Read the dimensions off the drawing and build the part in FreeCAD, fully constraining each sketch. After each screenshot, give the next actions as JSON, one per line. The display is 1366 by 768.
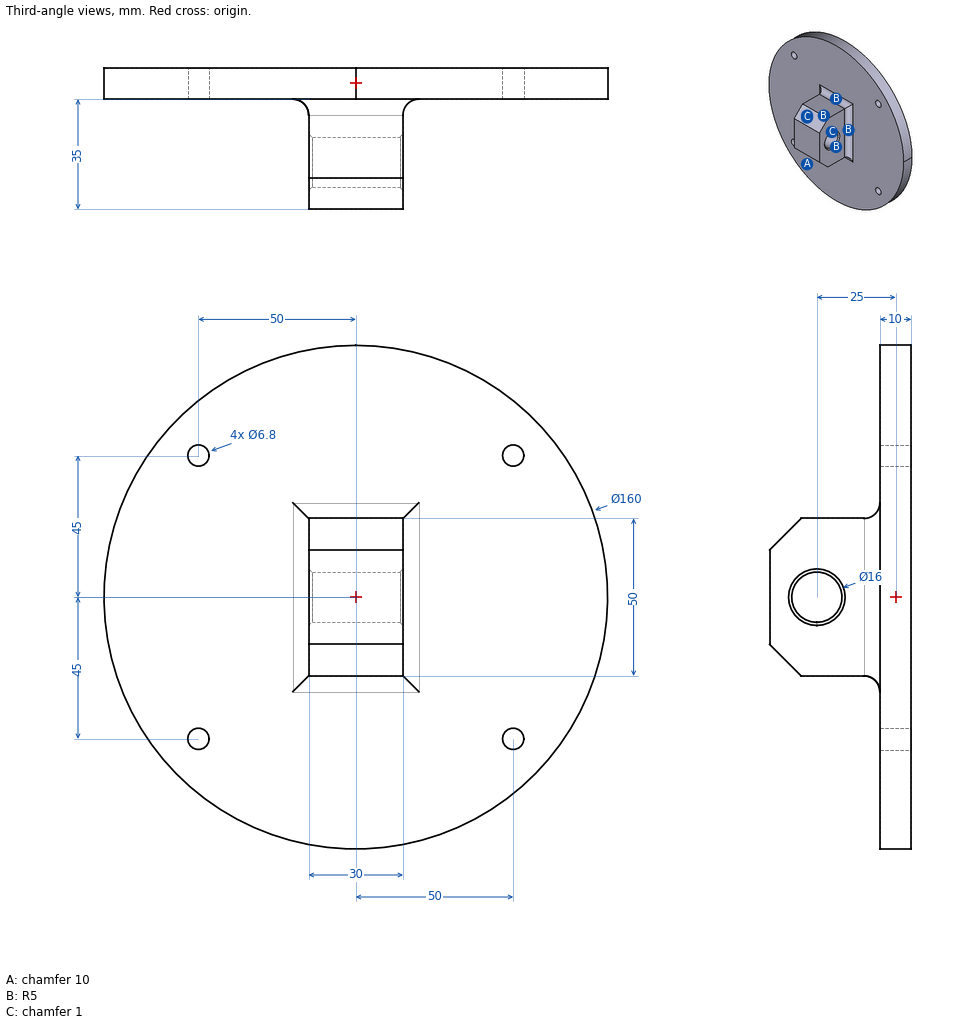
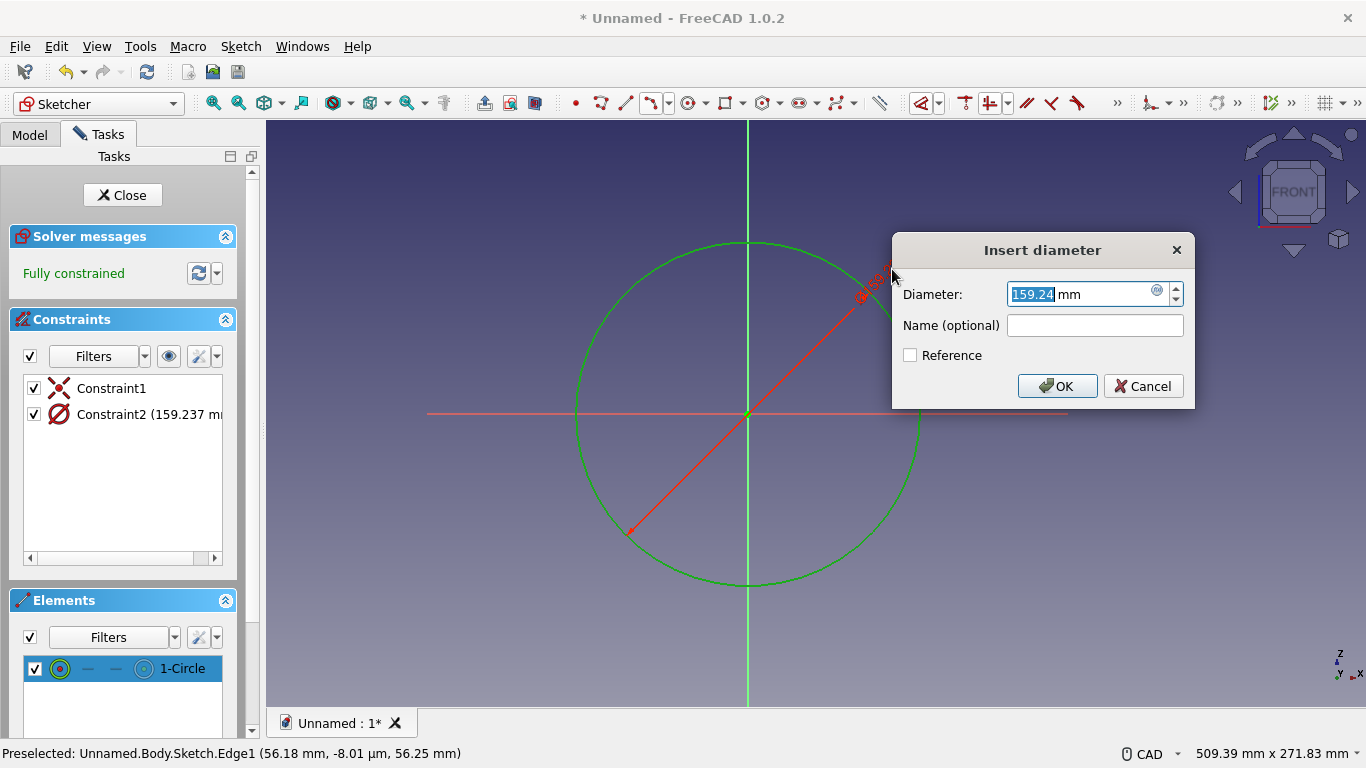
{"action": "type", "text": "160"}
{"action": "key", "text": "Return"}
{"action": "key", "text": "Escape"}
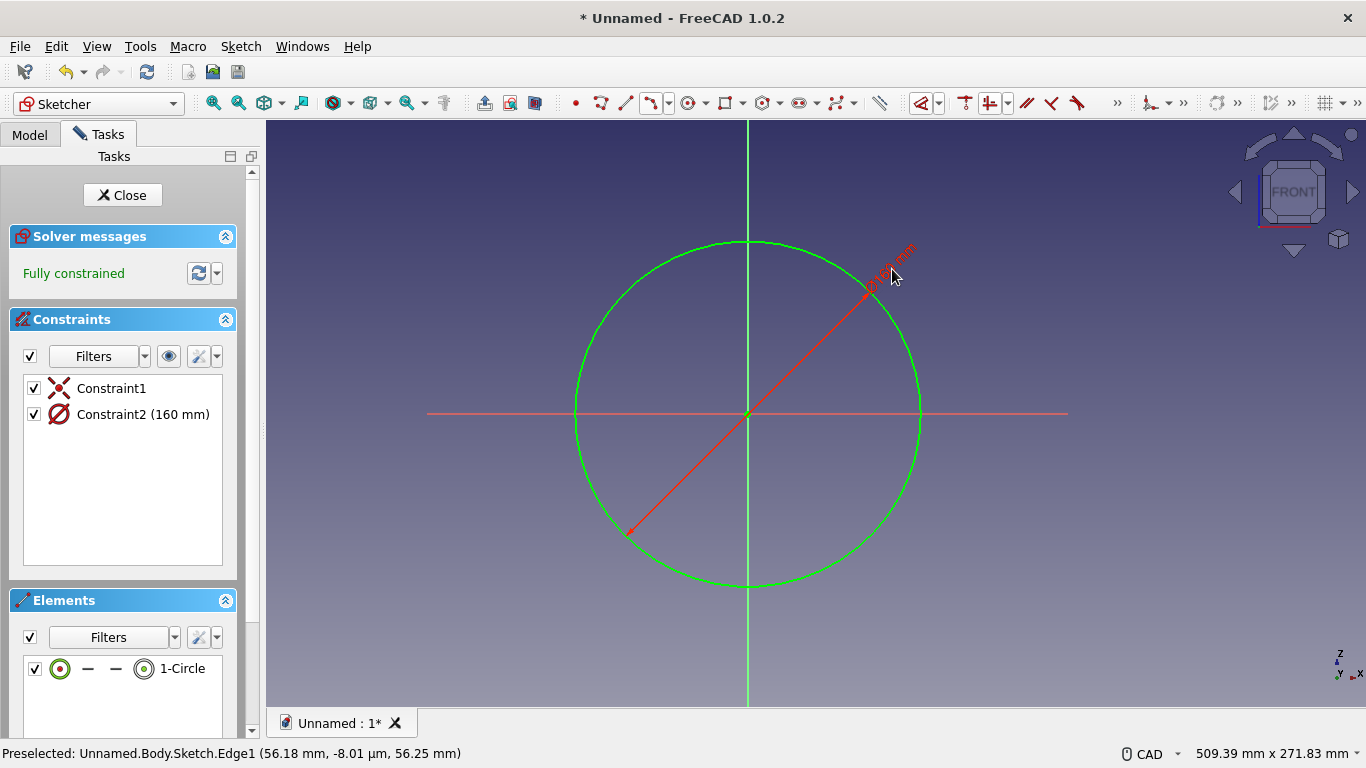
{"action": "left_click", "coordinate": [123, 195]}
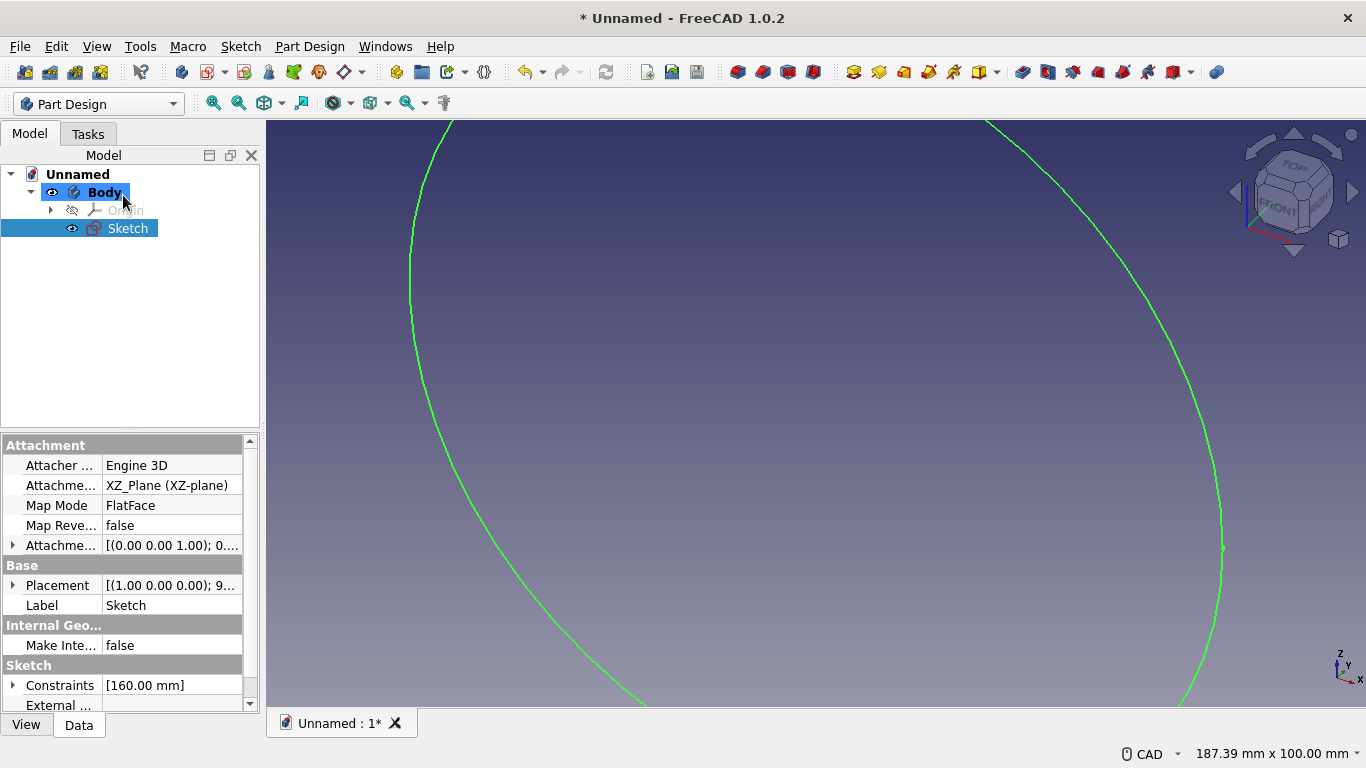
{"action": "left_click", "coordinate": [854, 72]}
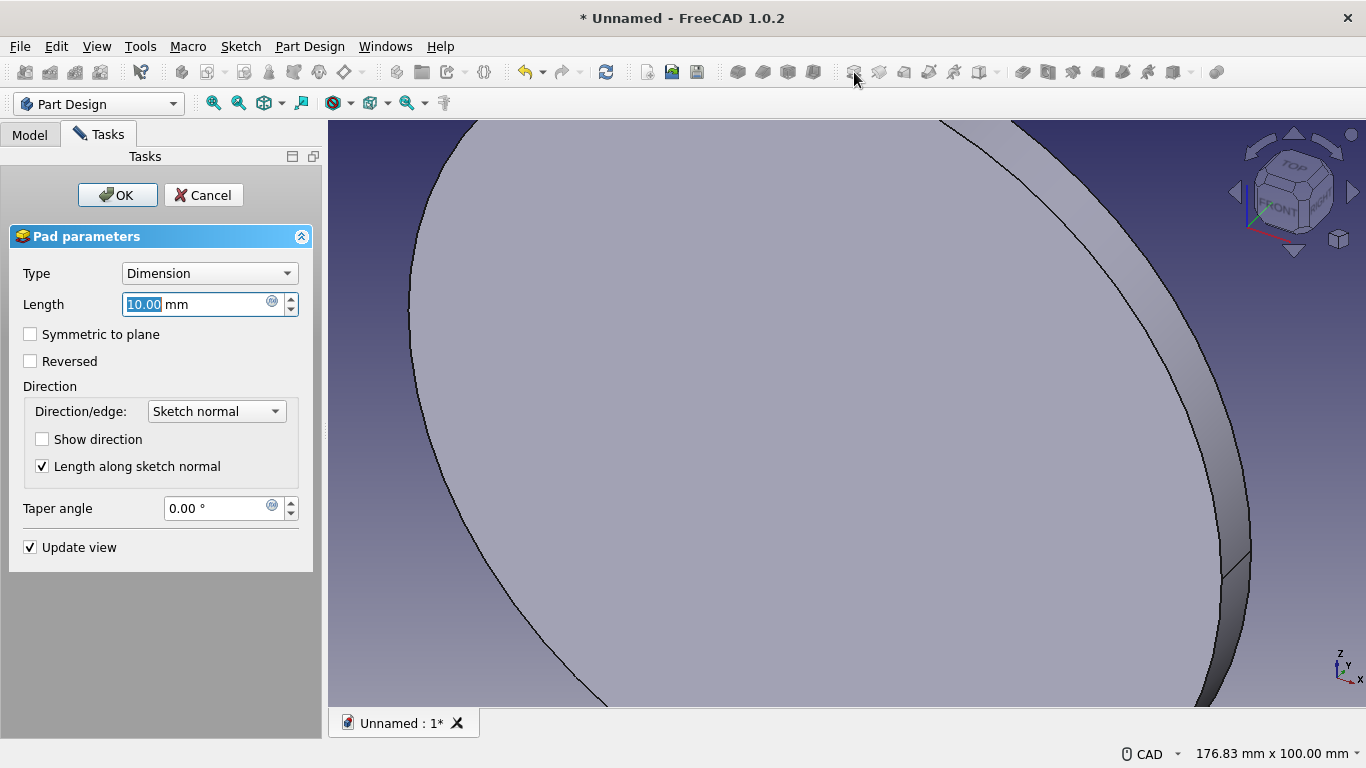
{"action": "type", "text": "10"}
{"action": "key", "text": "Tab"}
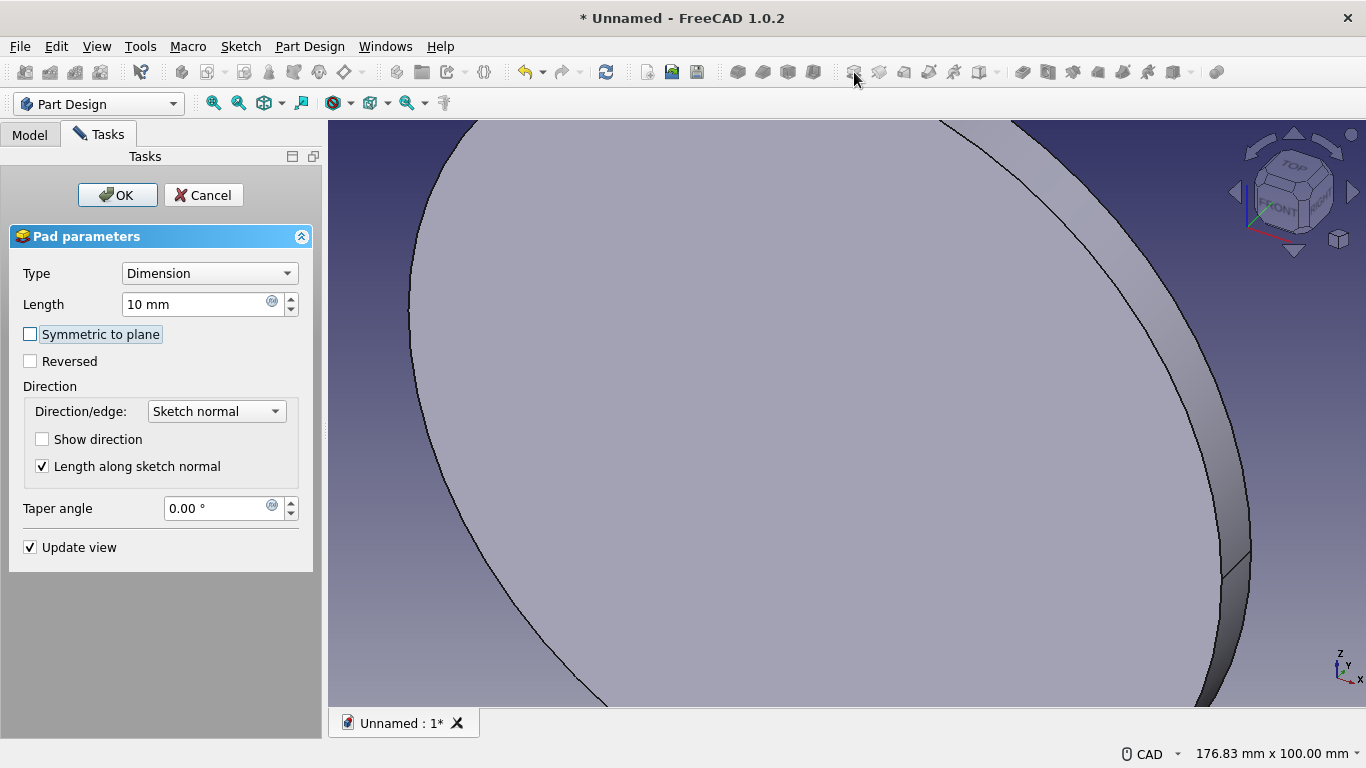
{"action": "left_click", "coordinate": [31, 334]}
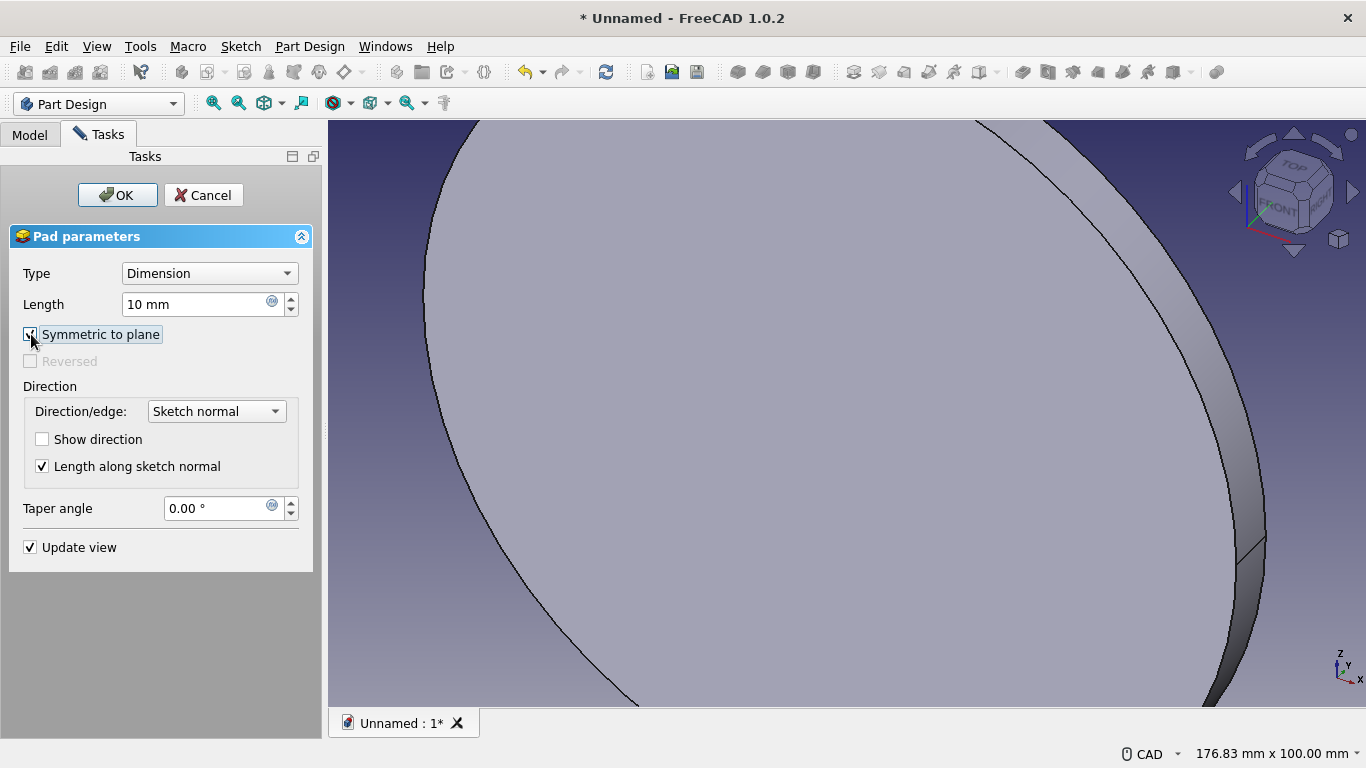
{"action": "left_click", "coordinate": [118, 195]}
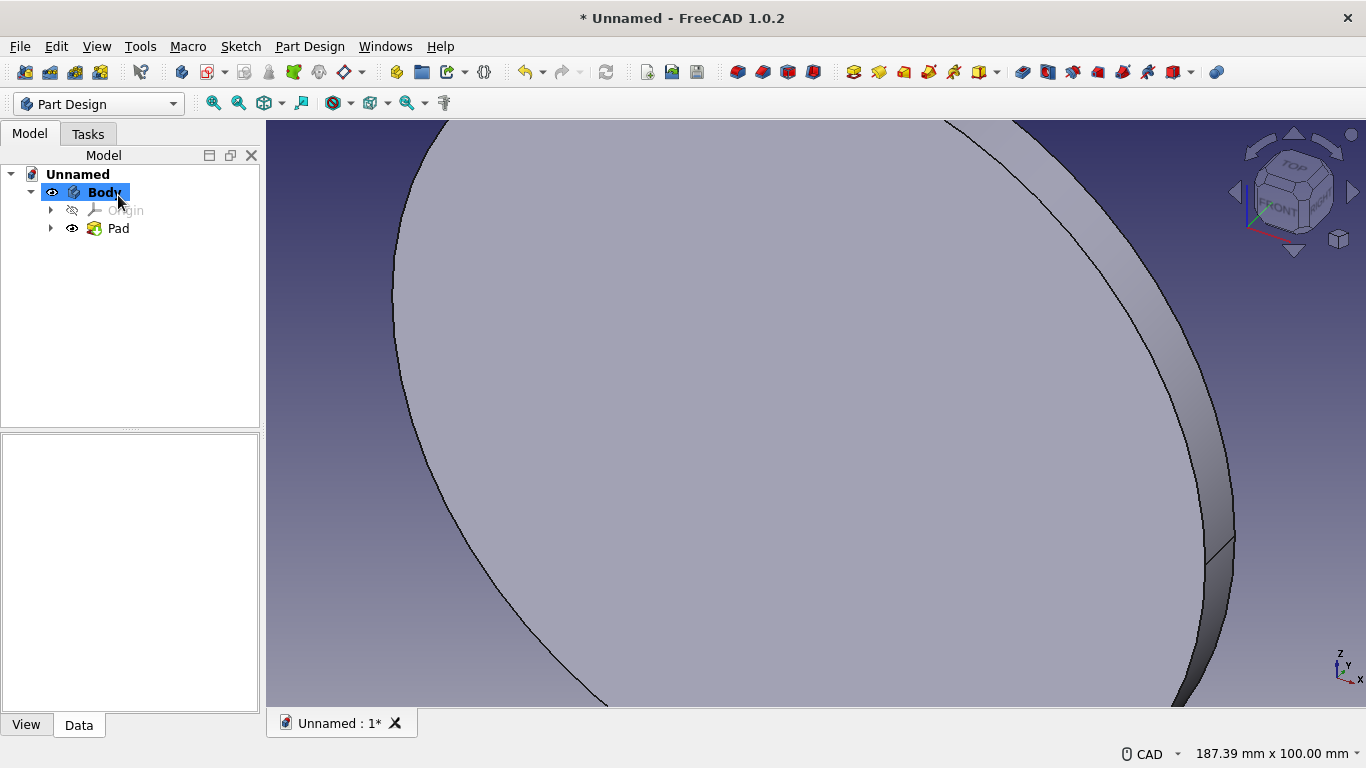
{"action": "key", "text": "v f"}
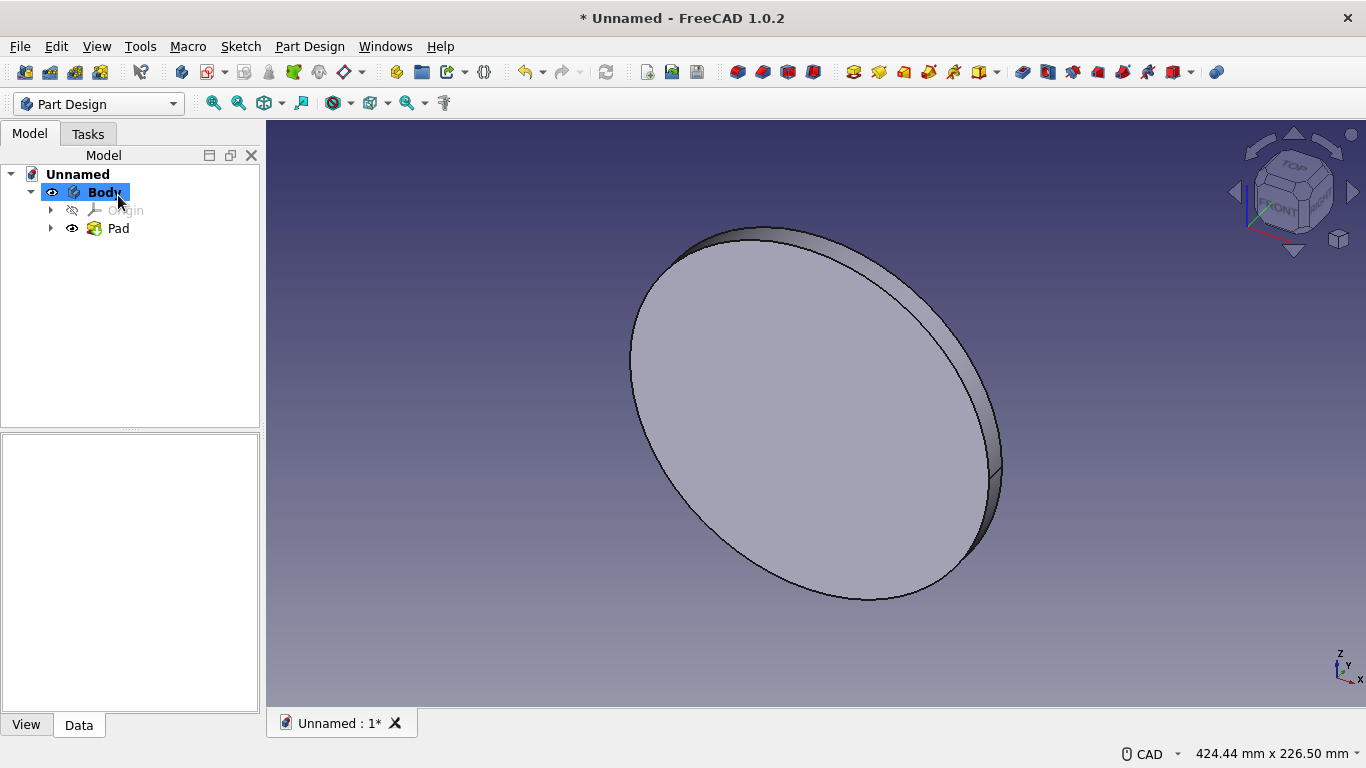
{"action": "left_click", "coordinate": [810, 419]}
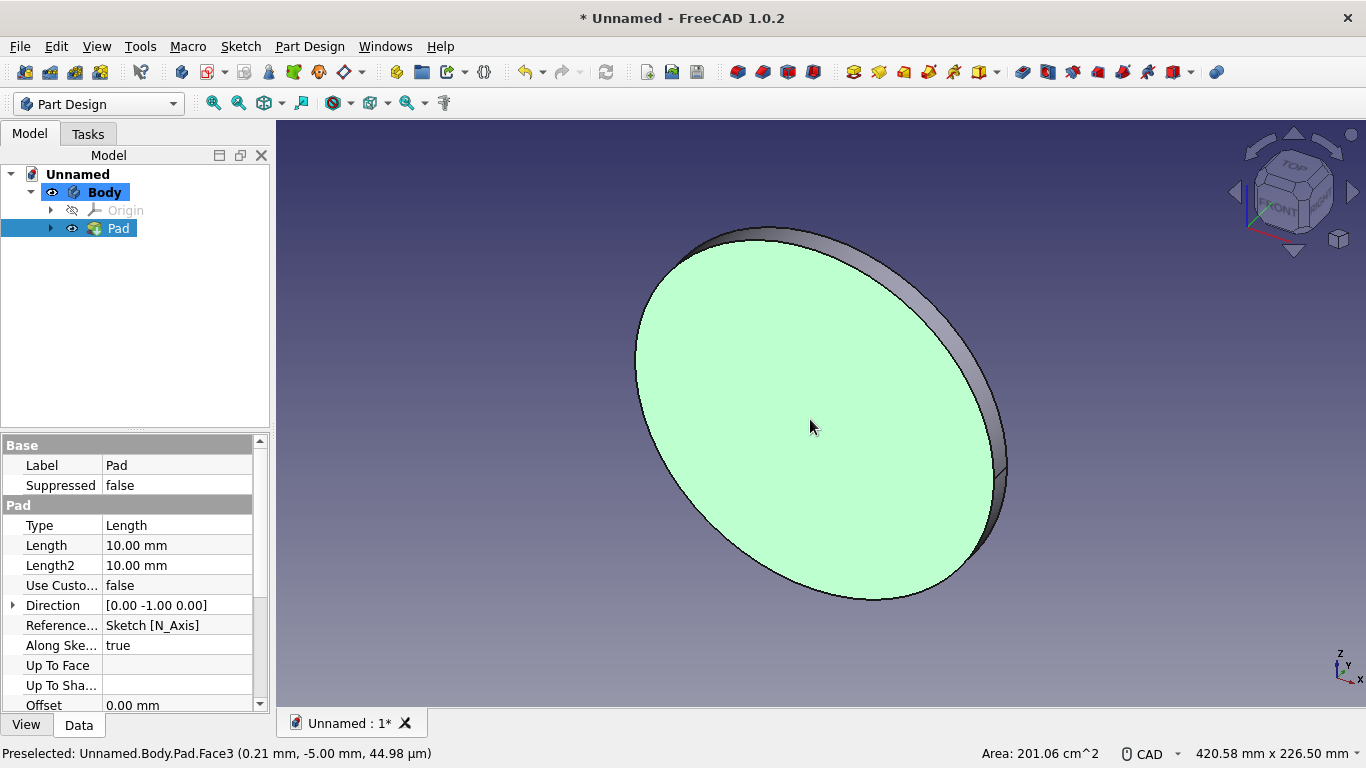
{"action": "left_click", "coordinate": [206, 72]}